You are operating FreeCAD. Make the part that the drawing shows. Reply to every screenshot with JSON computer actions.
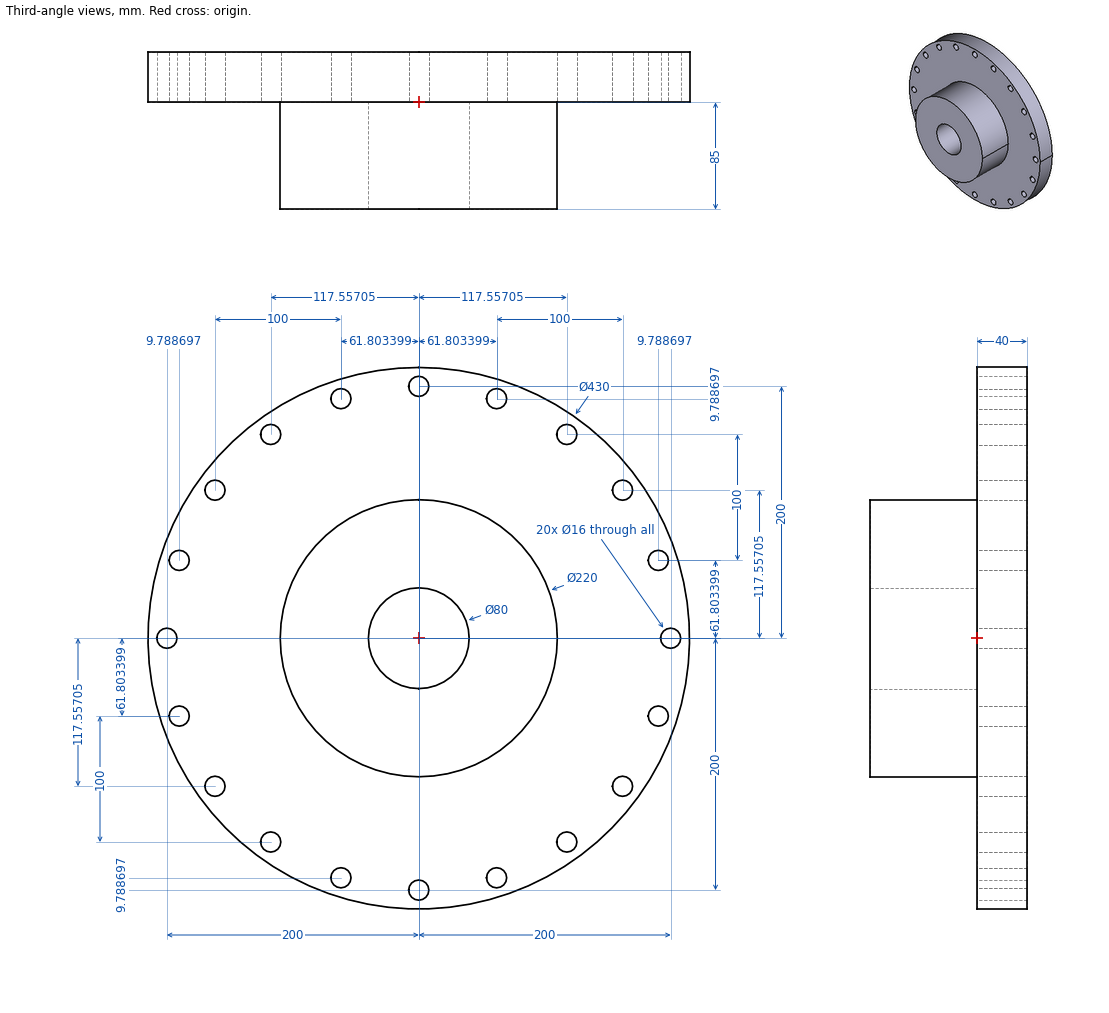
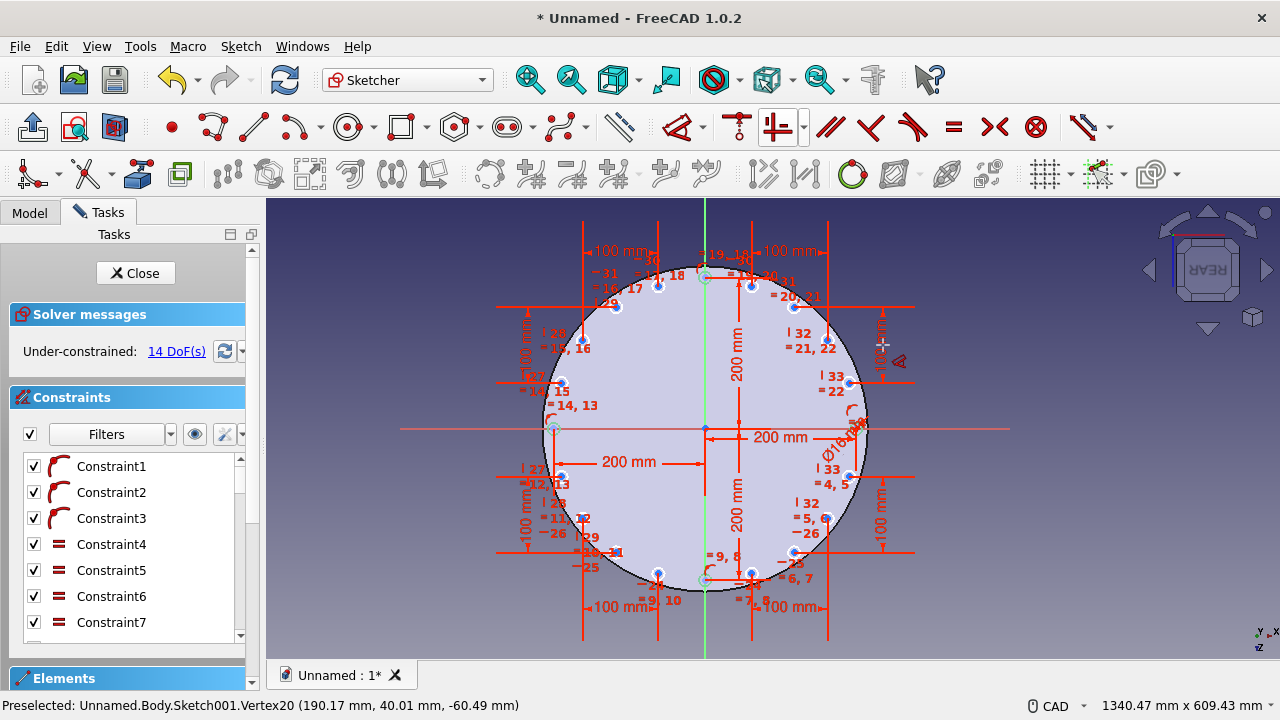
{"action": "left_click", "coordinate": [849, 477]}
{"action": "left_click", "coordinate": [883, 464]}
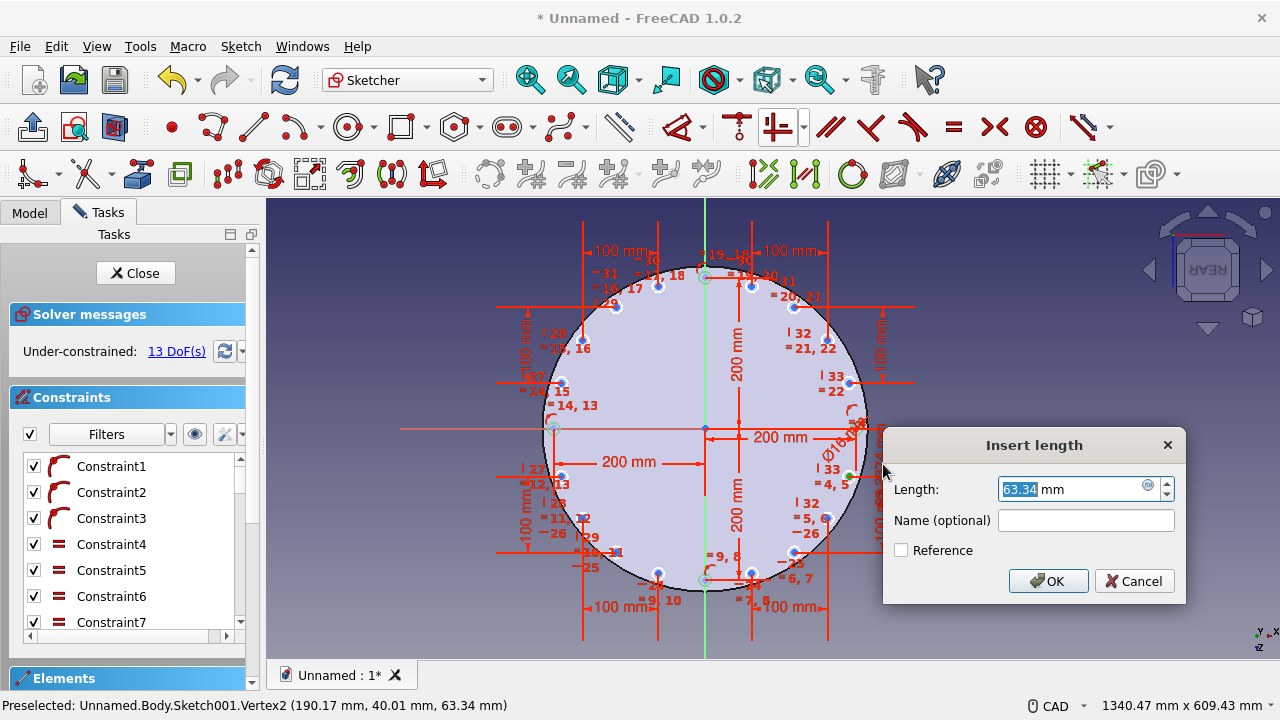
{"action": "type", "text": "61.803399"}
{"action": "key", "text": "Return"}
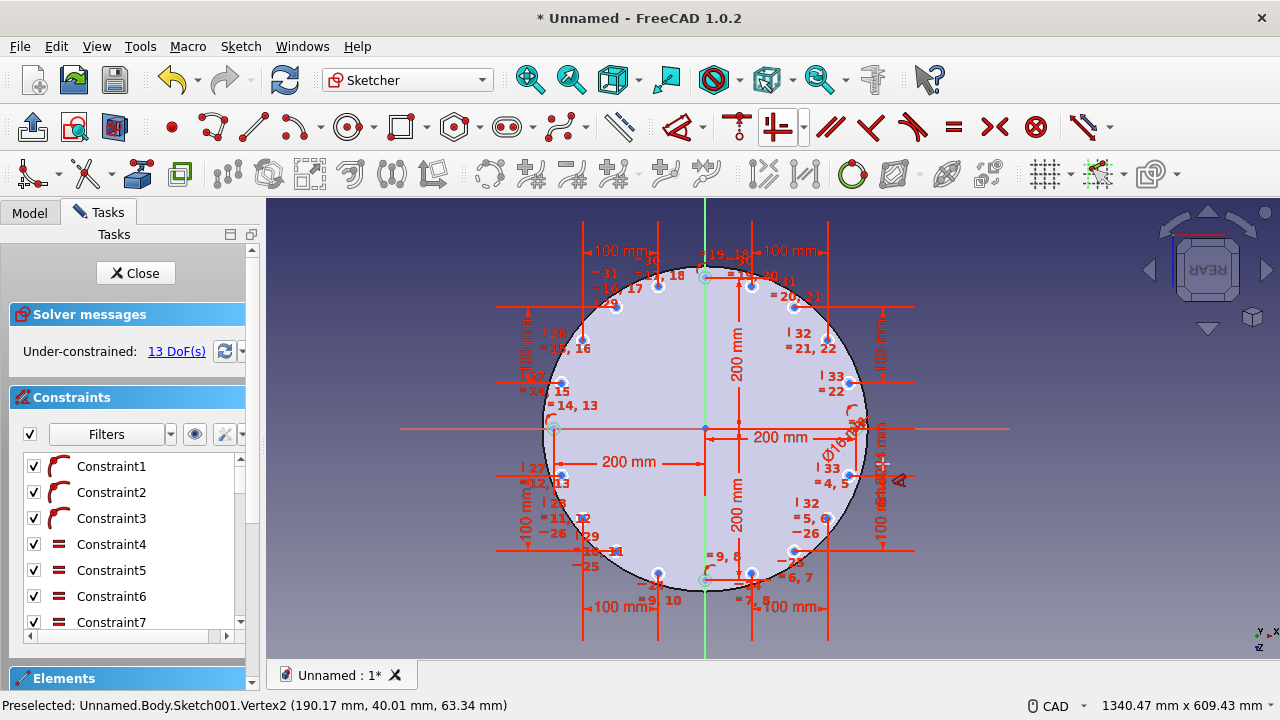
{"action": "left_click", "coordinate": [828, 519]}
{"action": "left_click", "coordinate": [862, 494]}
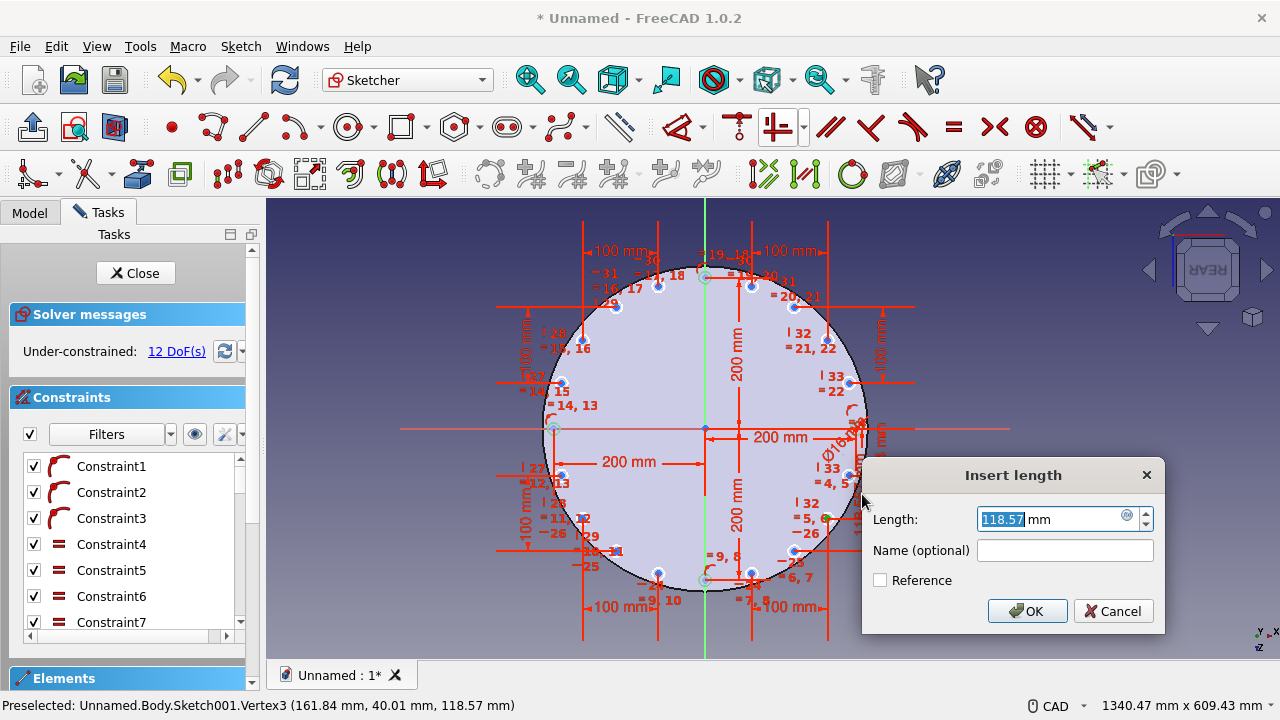
{"action": "type", "text": "117.55705"}
{"action": "key", "text": "Return"}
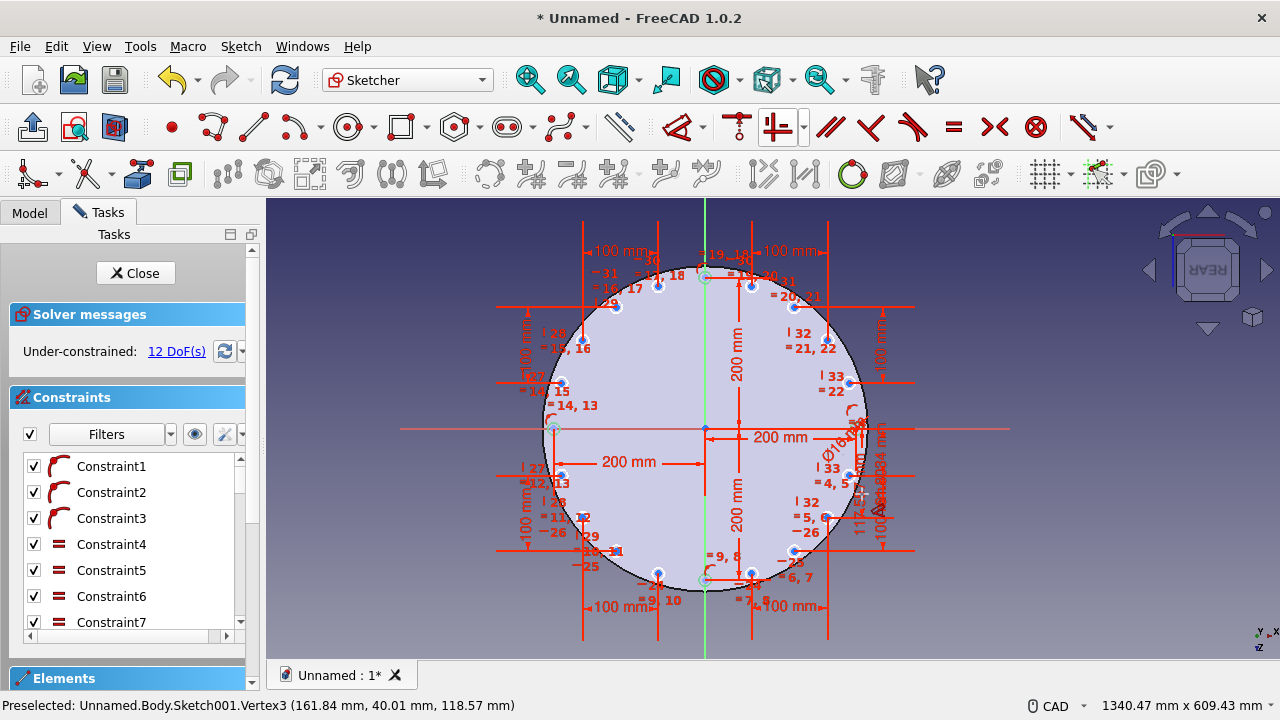
{"action": "left_click", "coordinate": [794, 551]}
{"action": "left_click", "coordinate": [729, 585]}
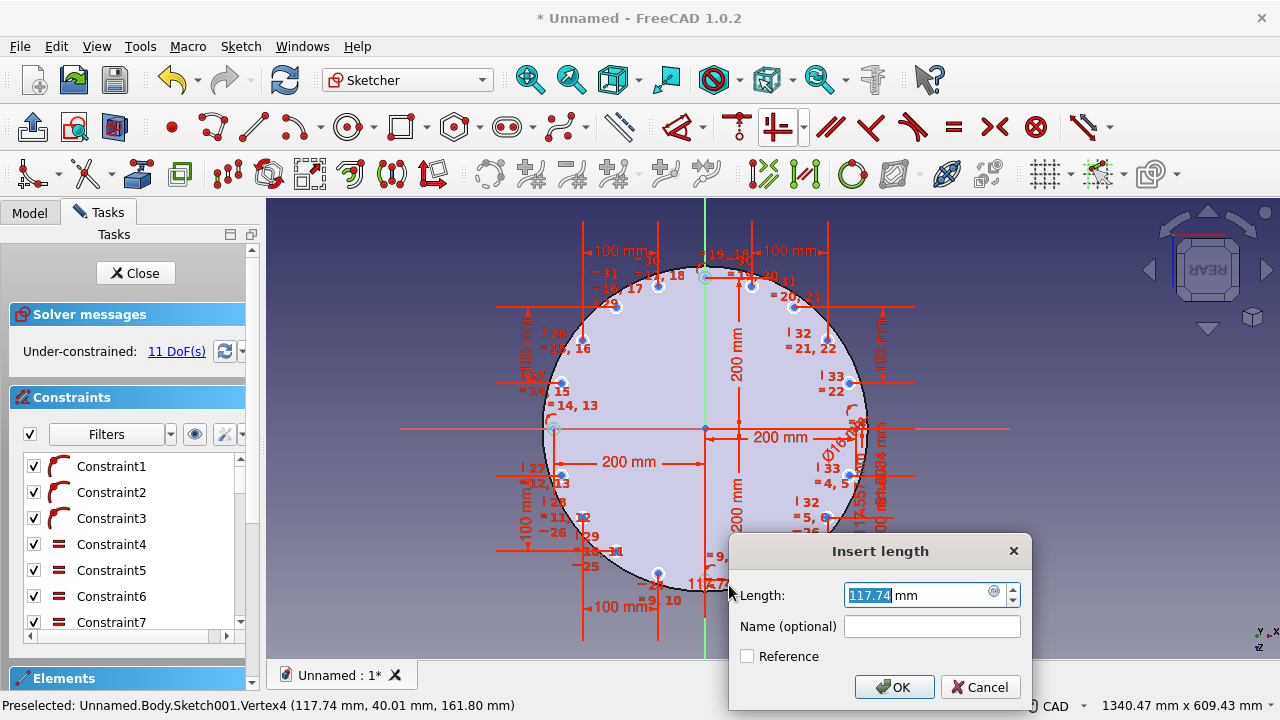
{"action": "type", "text": "117.55705"}
{"action": "key", "text": "Return"}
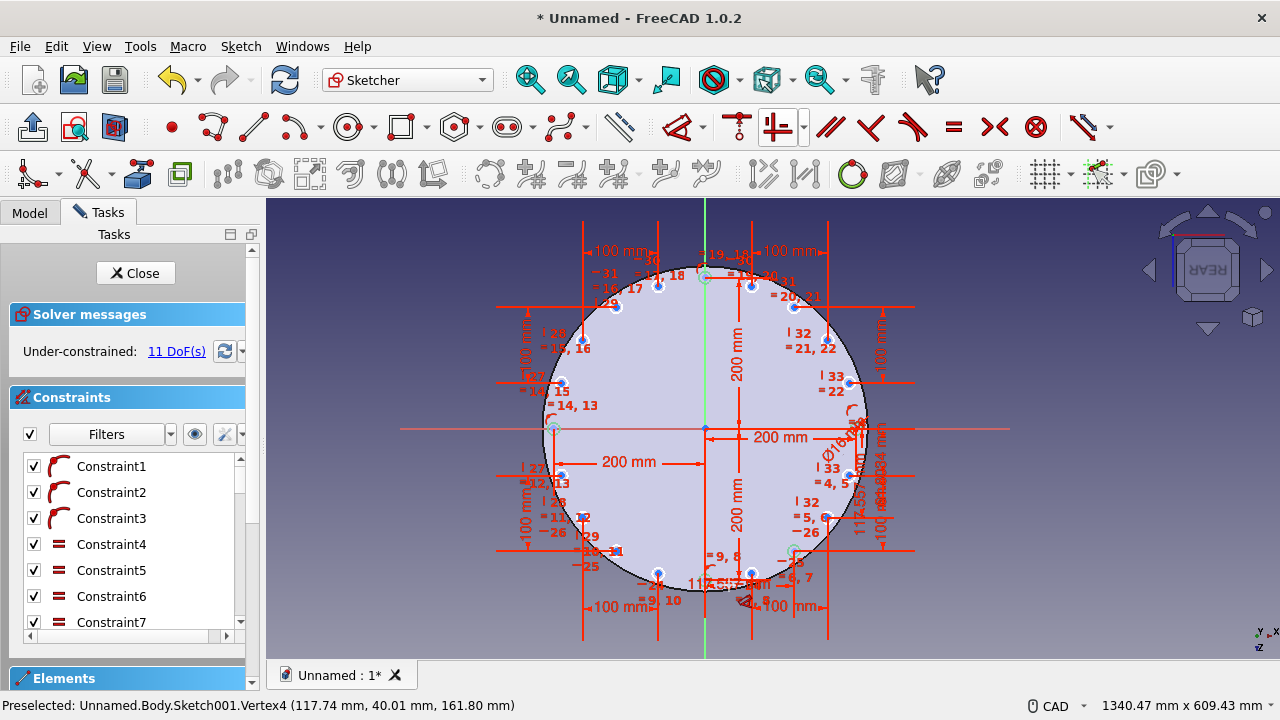
{"action": "left_click", "coordinate": [752, 574]}
{"action": "left_click", "coordinate": [729, 395]}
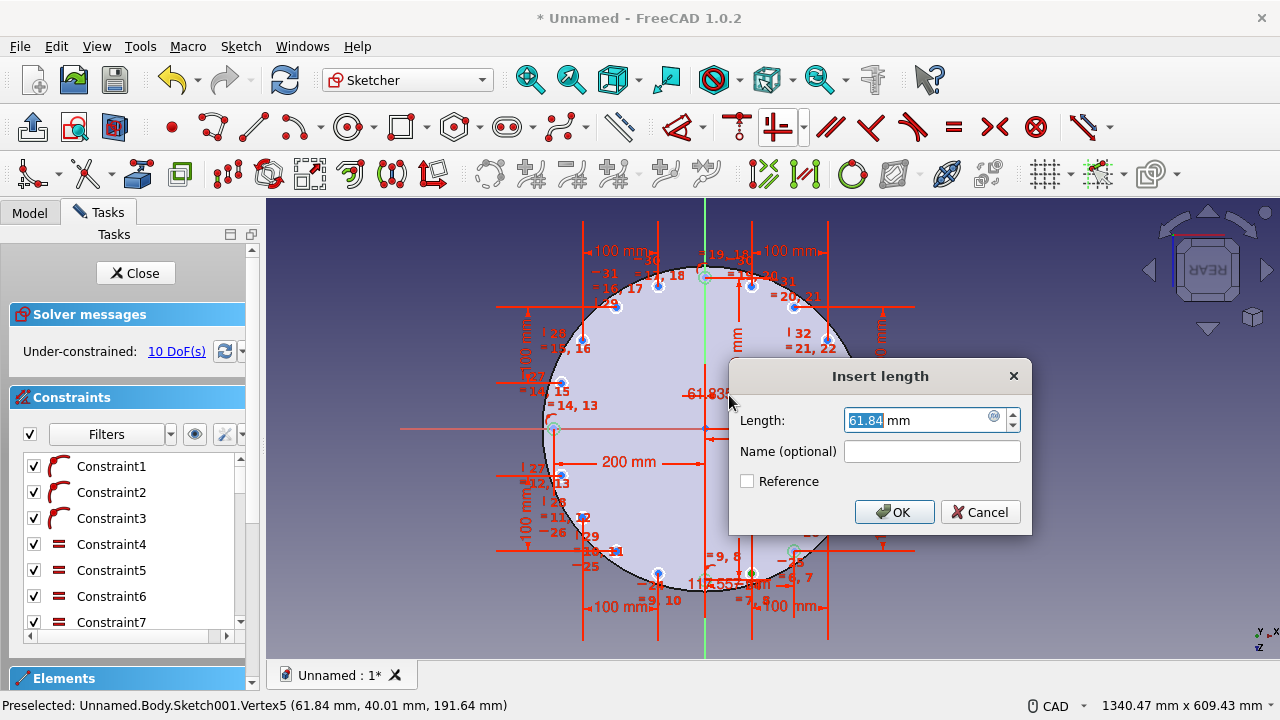
{"action": "type", "text": "61.803399"}
{"action": "key", "text": "Return"}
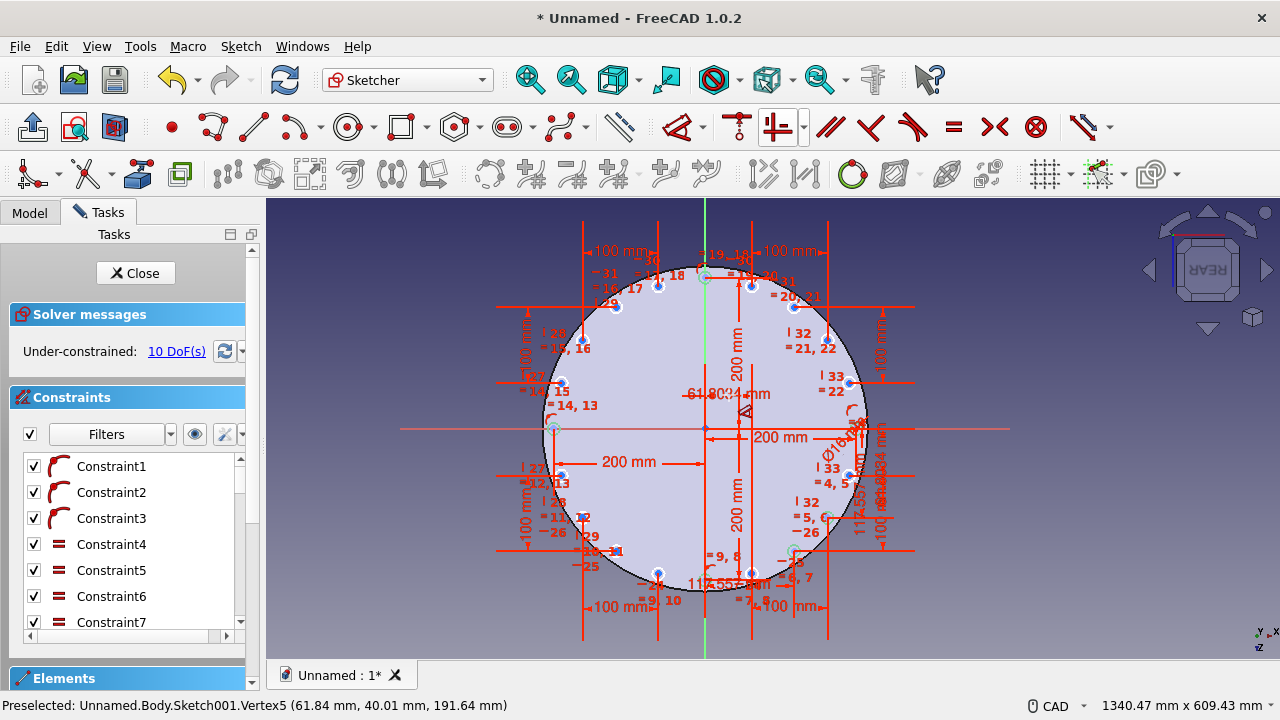
{"action": "left_click", "coordinate": [658, 574]}
{"action": "left_click", "coordinate": [665, 371]}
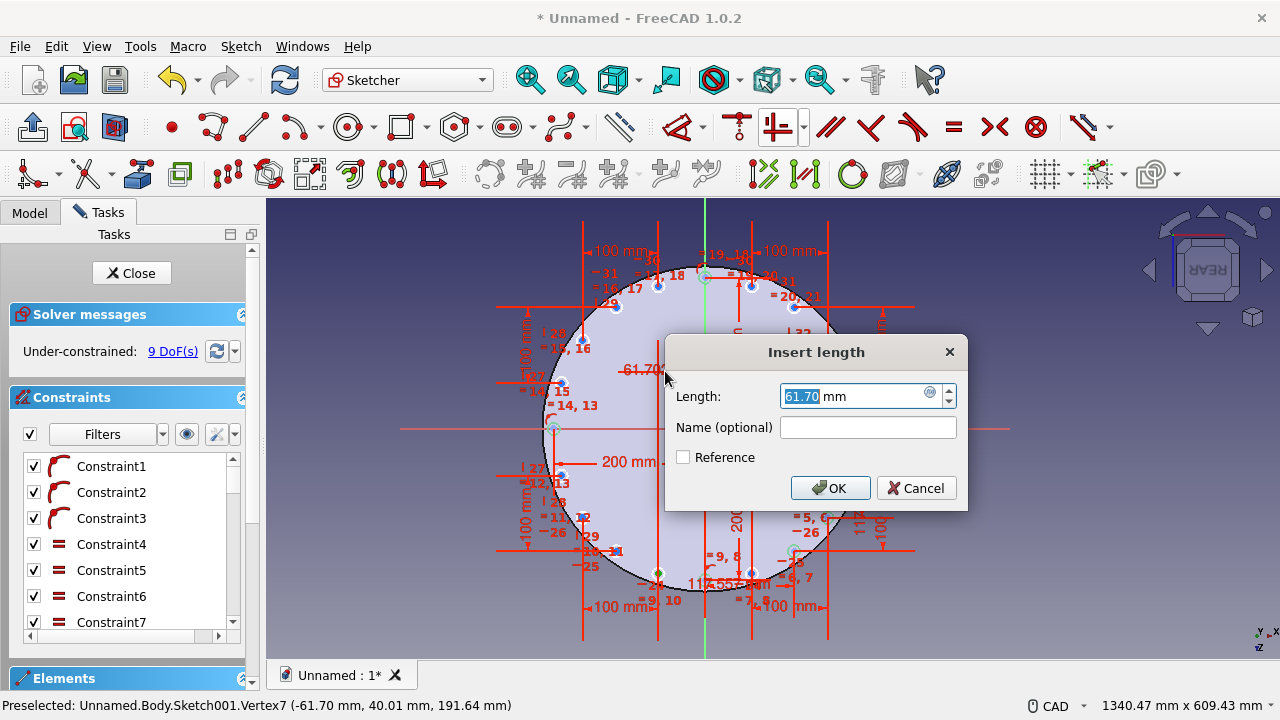
{"action": "type", "text": "61.803399"}
{"action": "key", "text": "Return"}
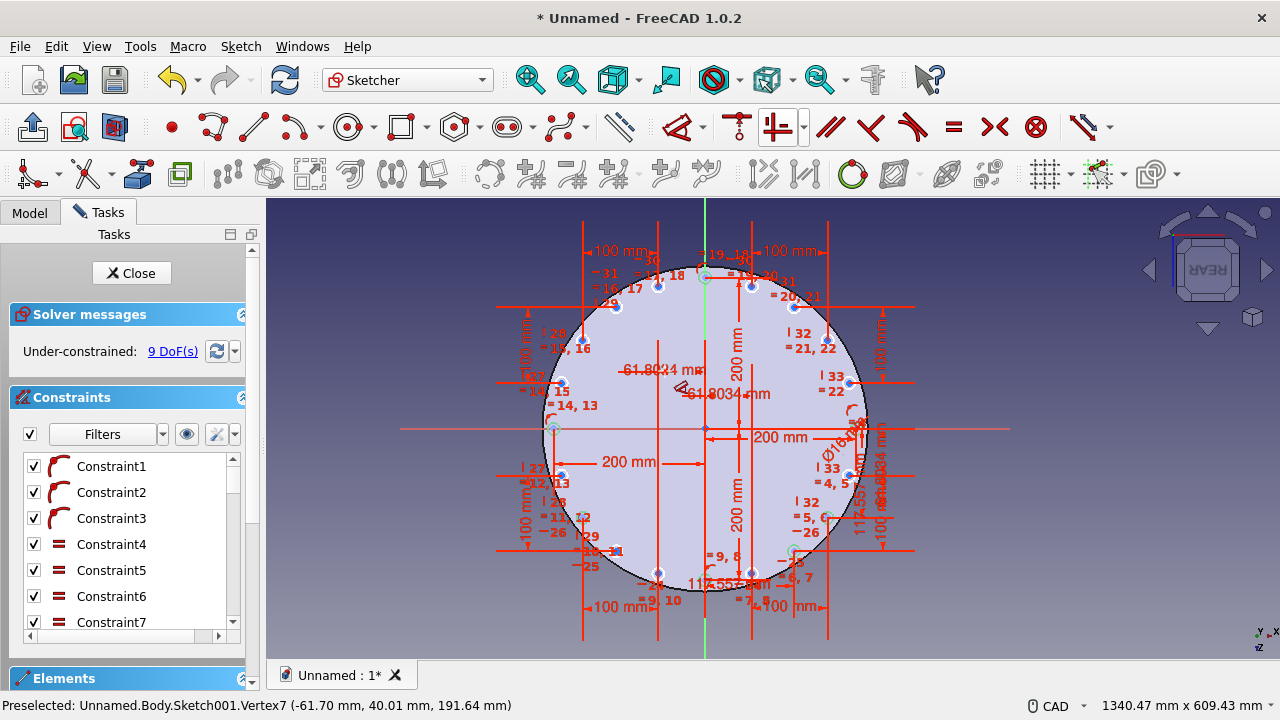
{"action": "left_click", "coordinate": [616, 551]}
{"action": "left_click", "coordinate": [640, 585]}